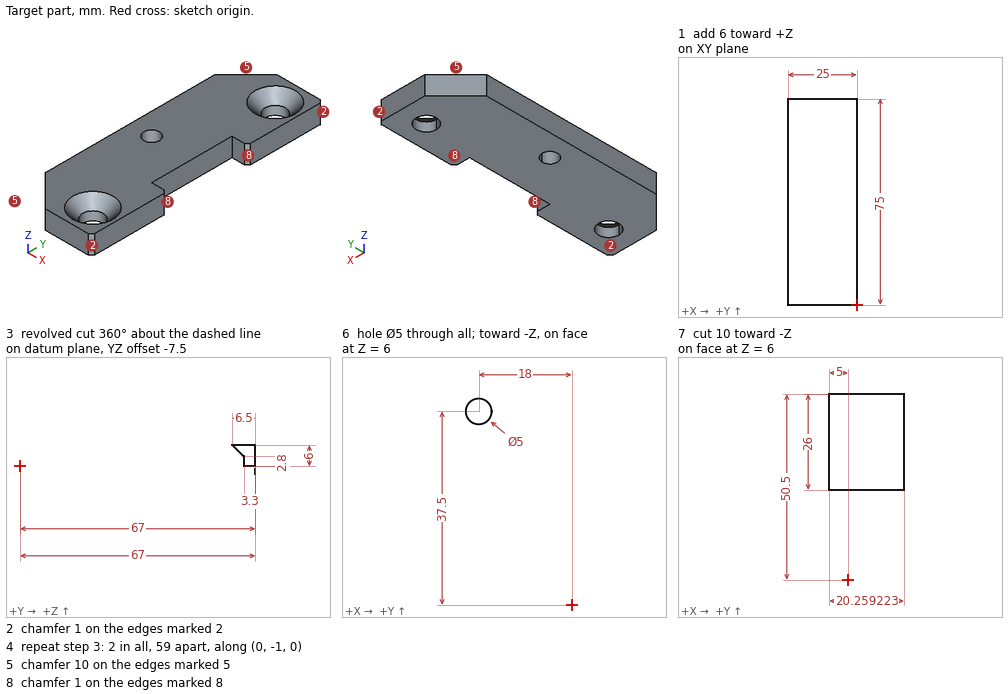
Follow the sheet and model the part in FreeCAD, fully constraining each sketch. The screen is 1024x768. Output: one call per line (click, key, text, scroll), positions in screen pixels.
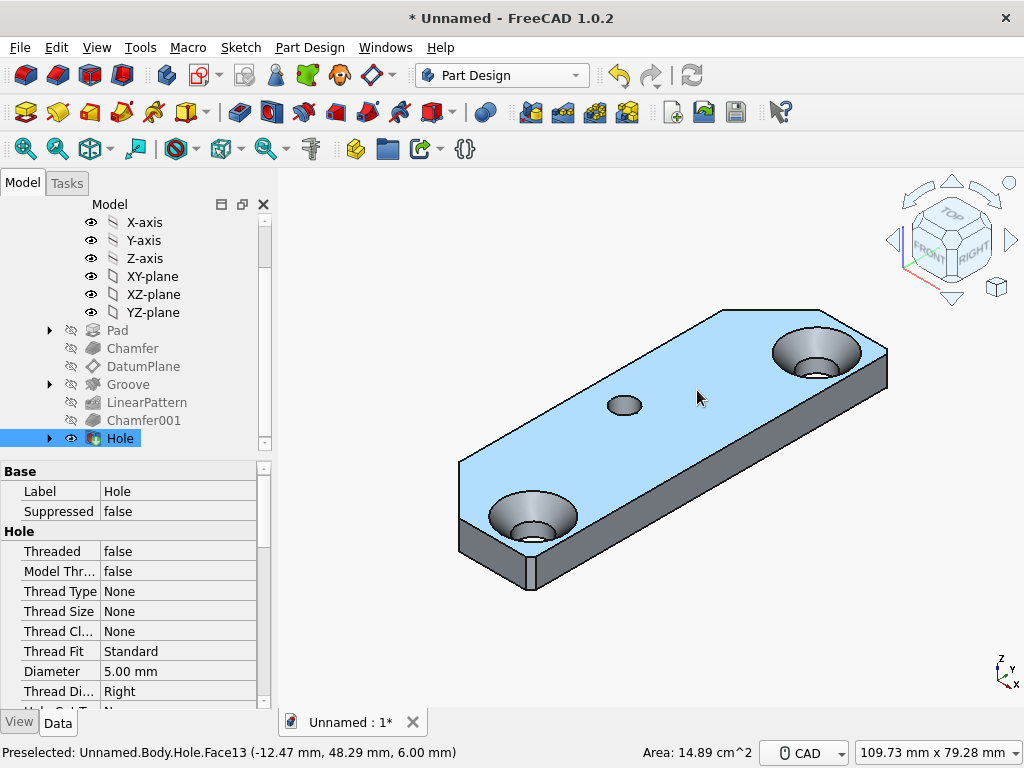
click(200, 76)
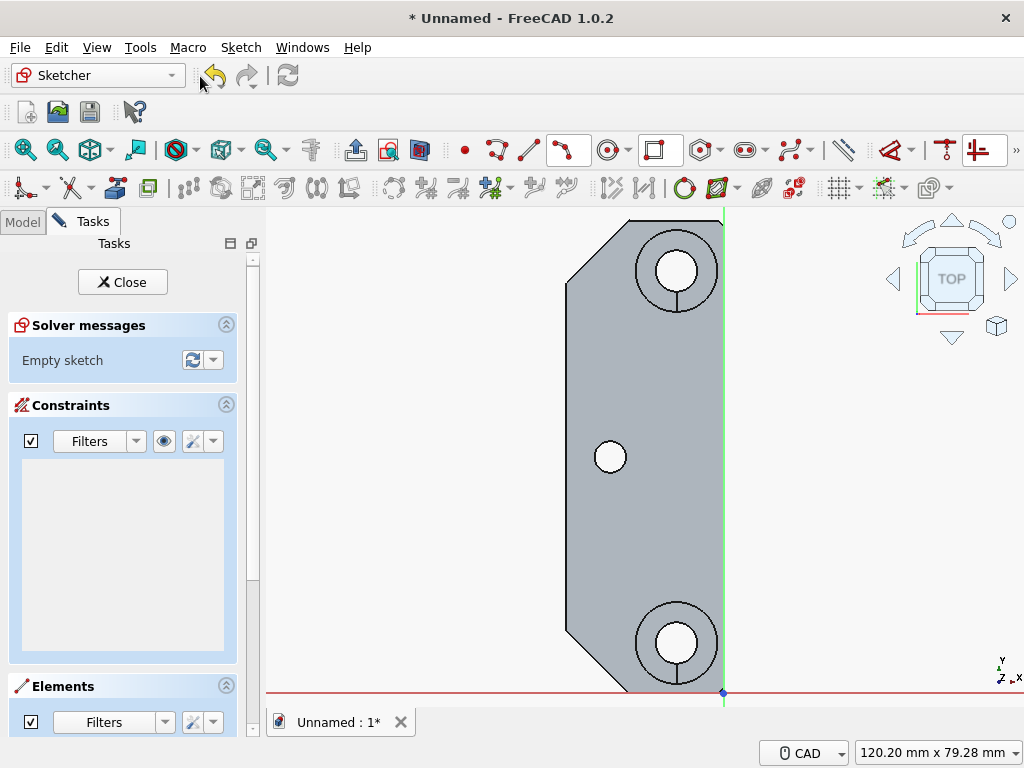
scroll(294, 235, down, 1)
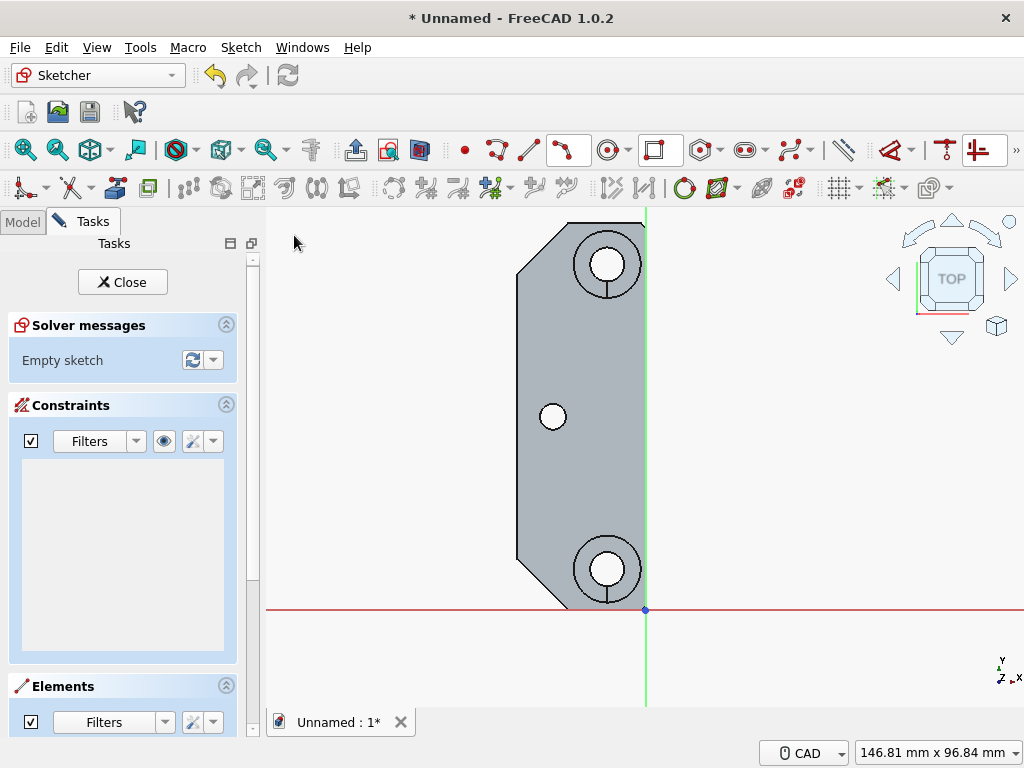
click(654, 150)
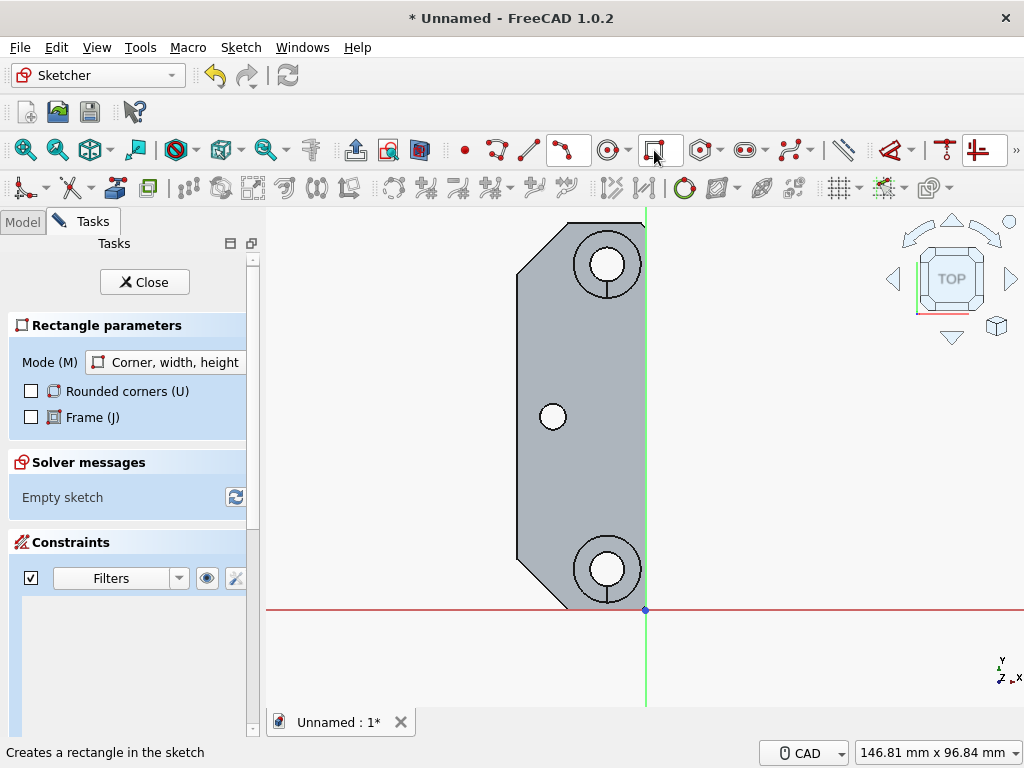
click(620, 350)
click(725, 484)
key(Escape)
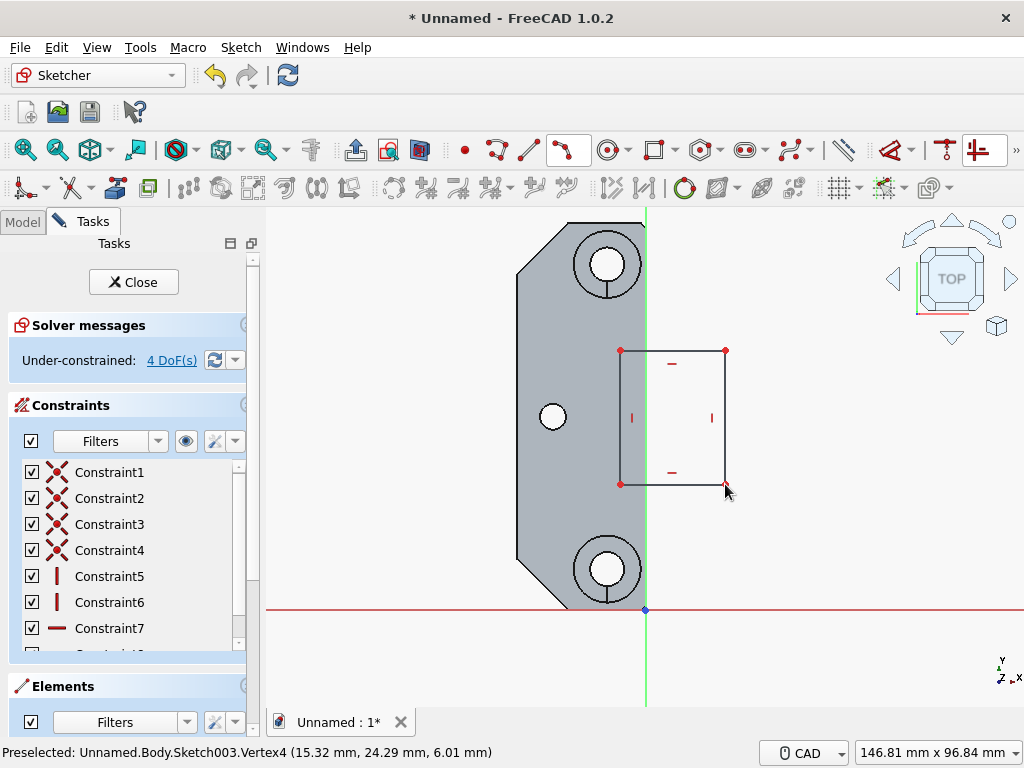
click(890, 150)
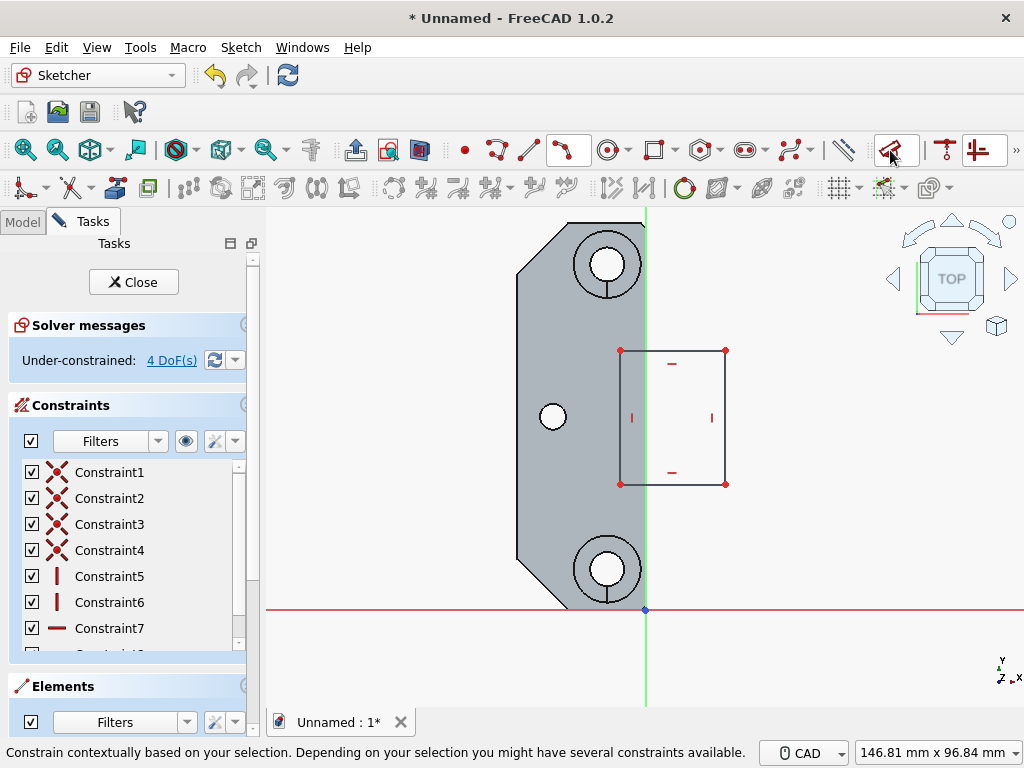
click(620, 391)
click(586, 418)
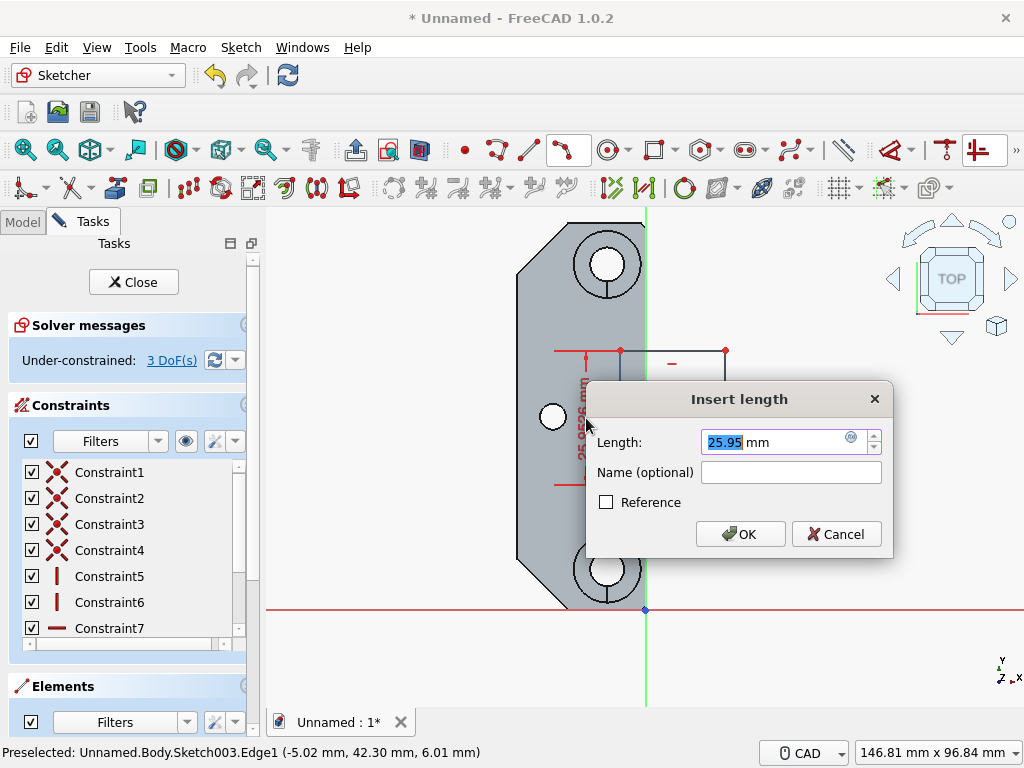
text(26)
key(Return)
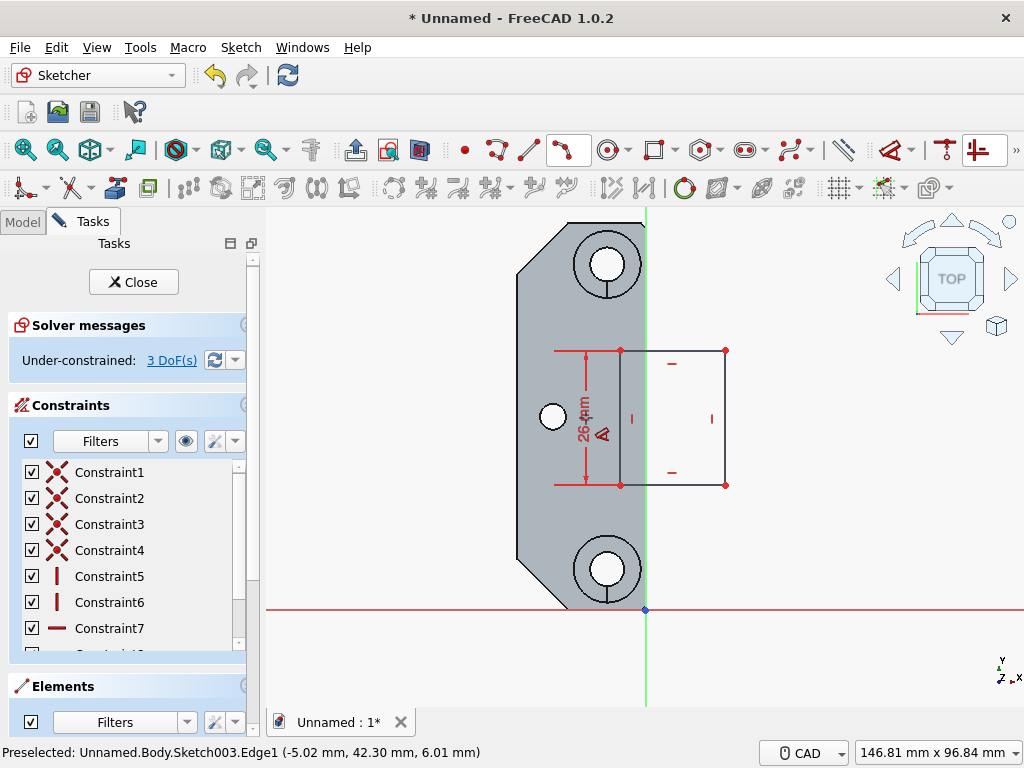
scroll(620, 351, up, 3)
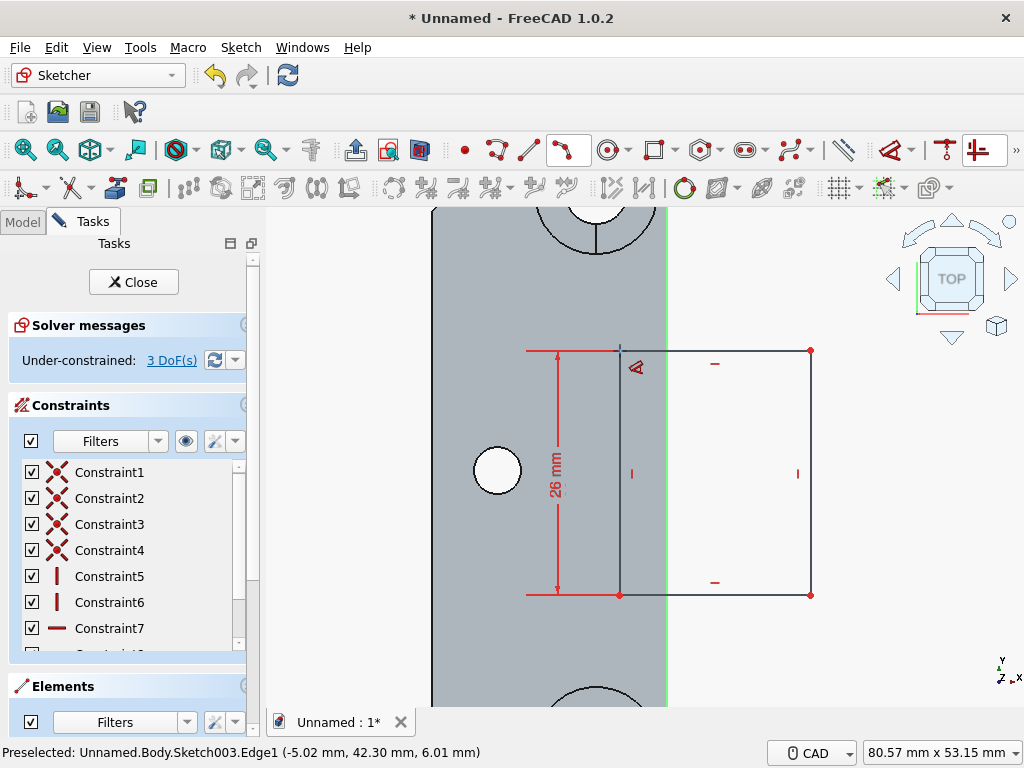
click(620, 351)
click(643, 317)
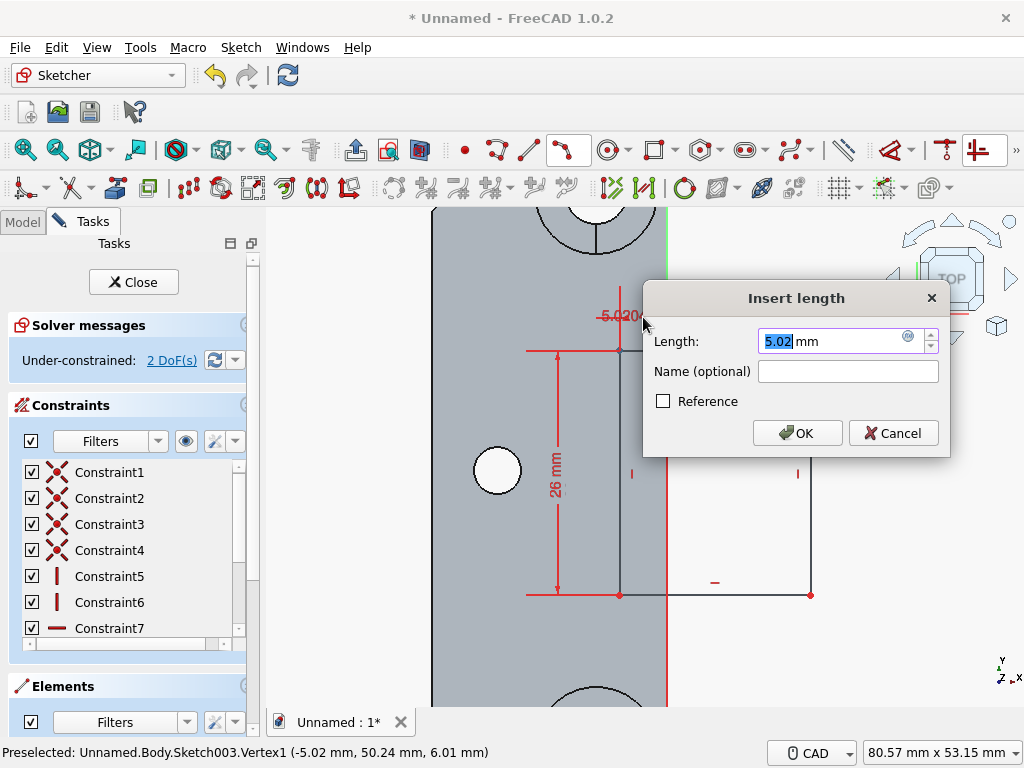
text(5)
key(Return)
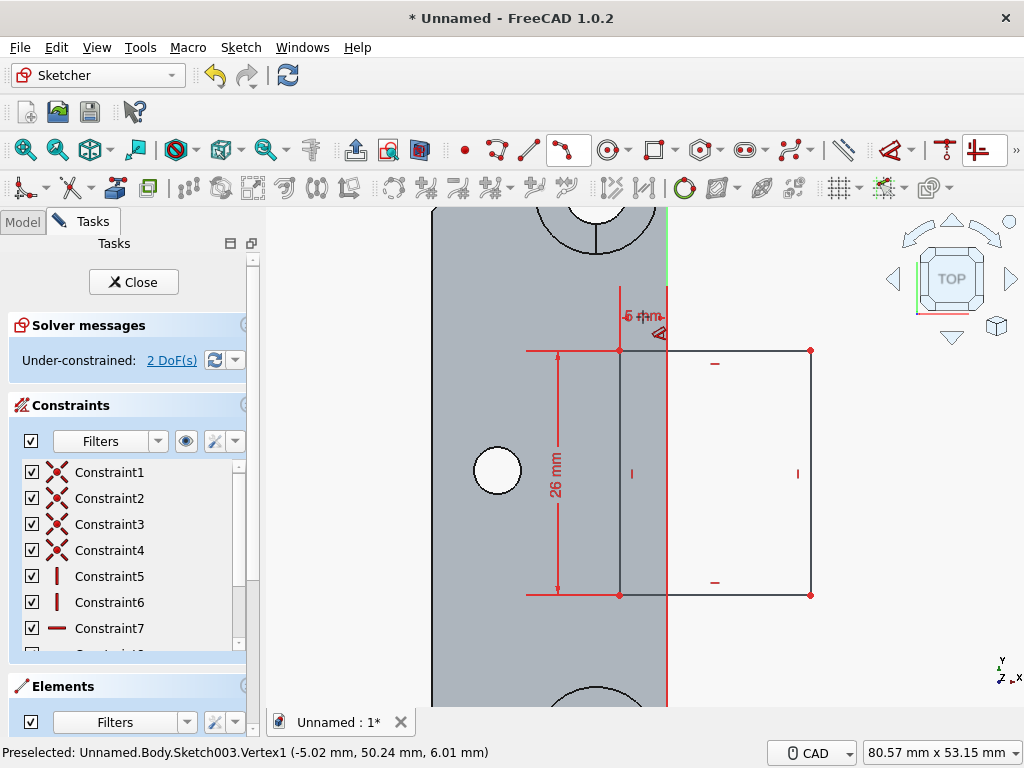
click(620, 351)
click(586, 515)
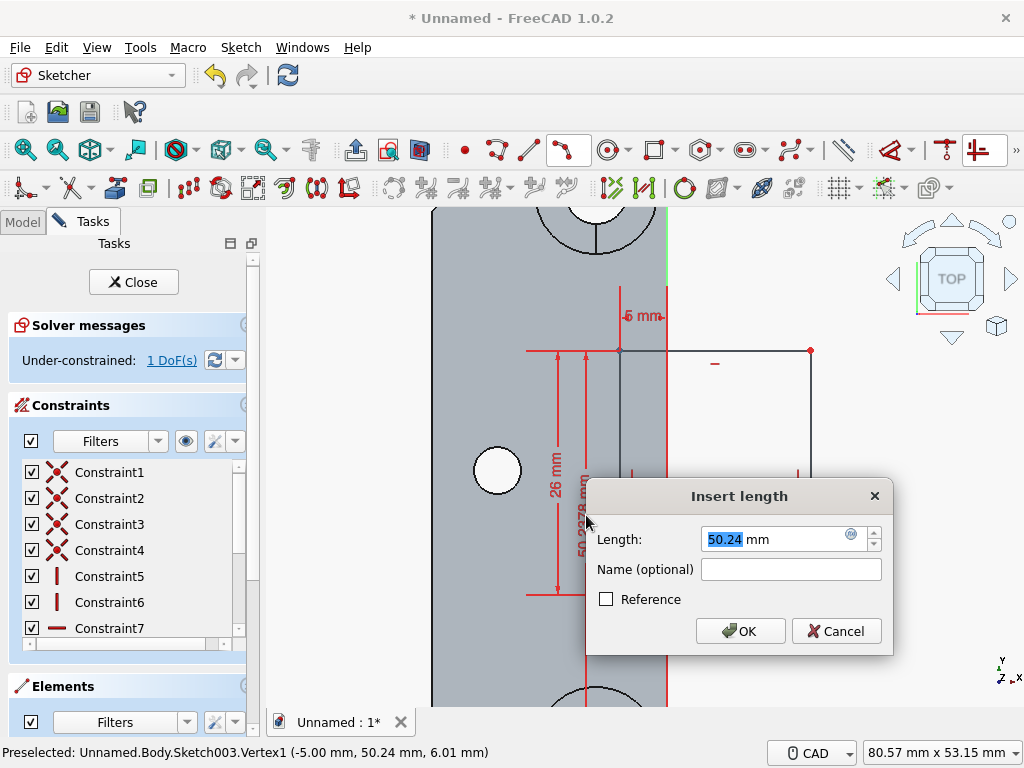
text(50.5)
key(Return)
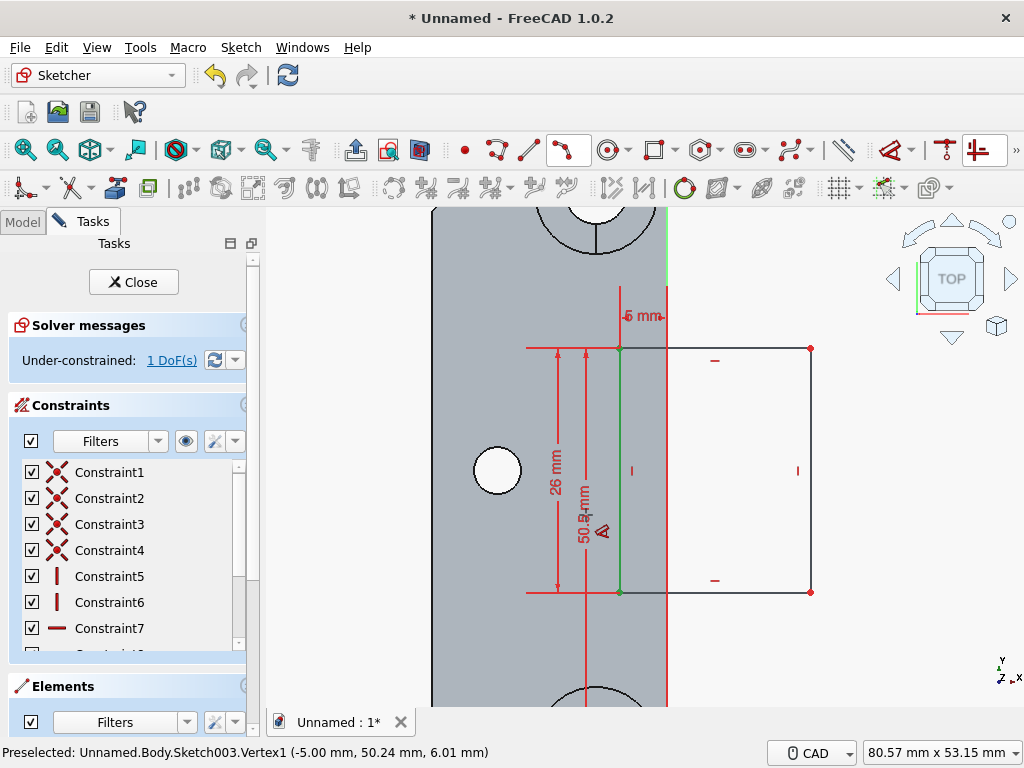
scroll(677, 593, up, 2)